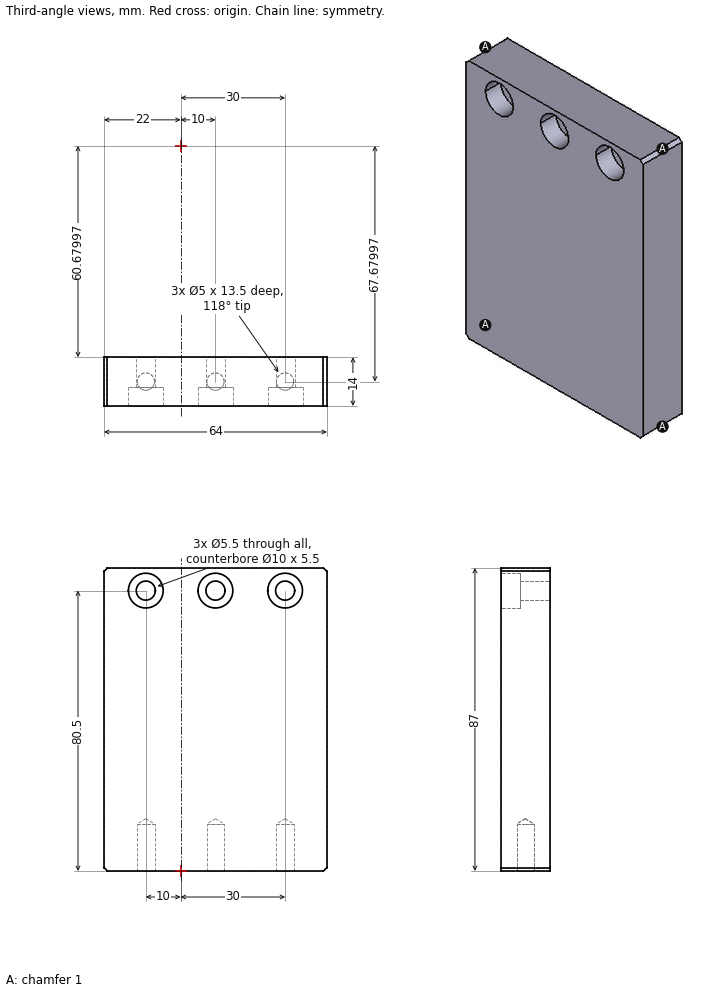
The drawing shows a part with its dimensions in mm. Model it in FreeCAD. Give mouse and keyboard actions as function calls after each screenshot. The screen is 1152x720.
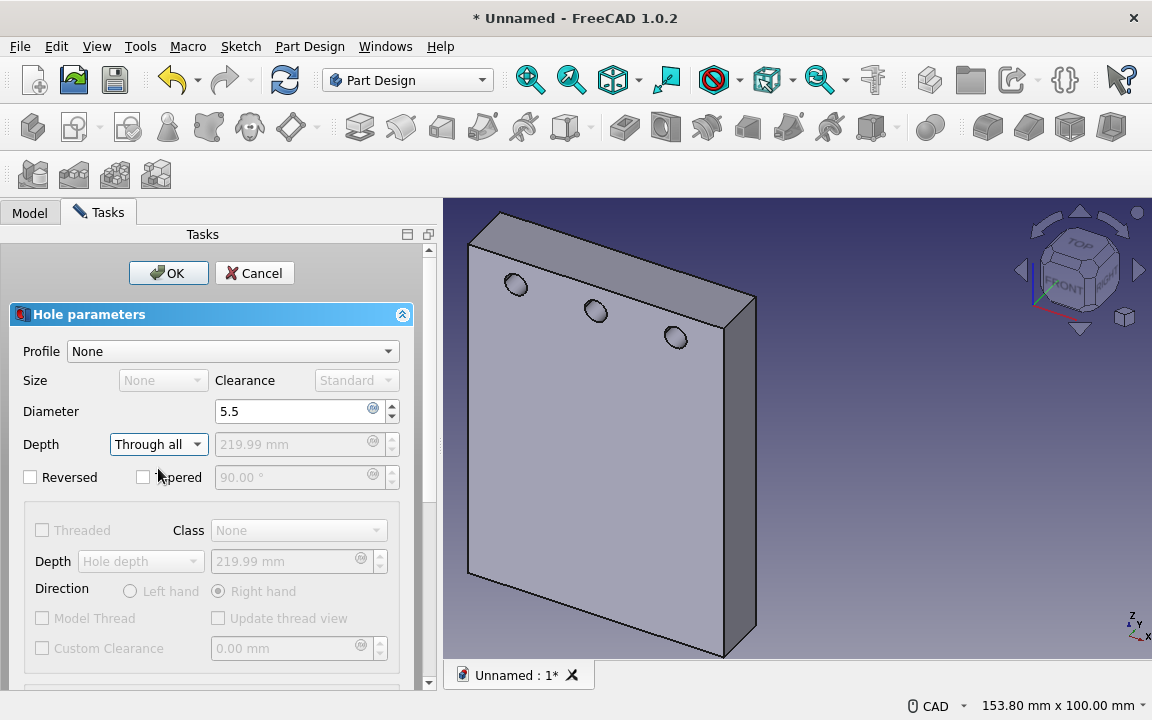
scroll(429, 467, down, 2)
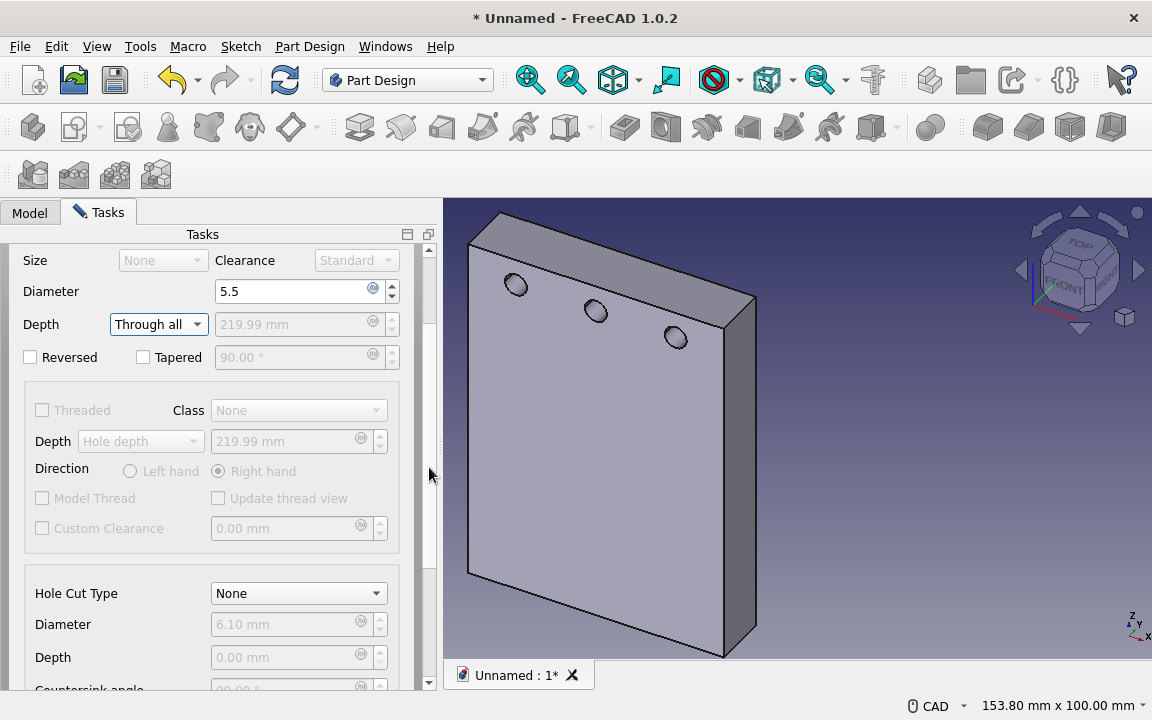
click(300, 594)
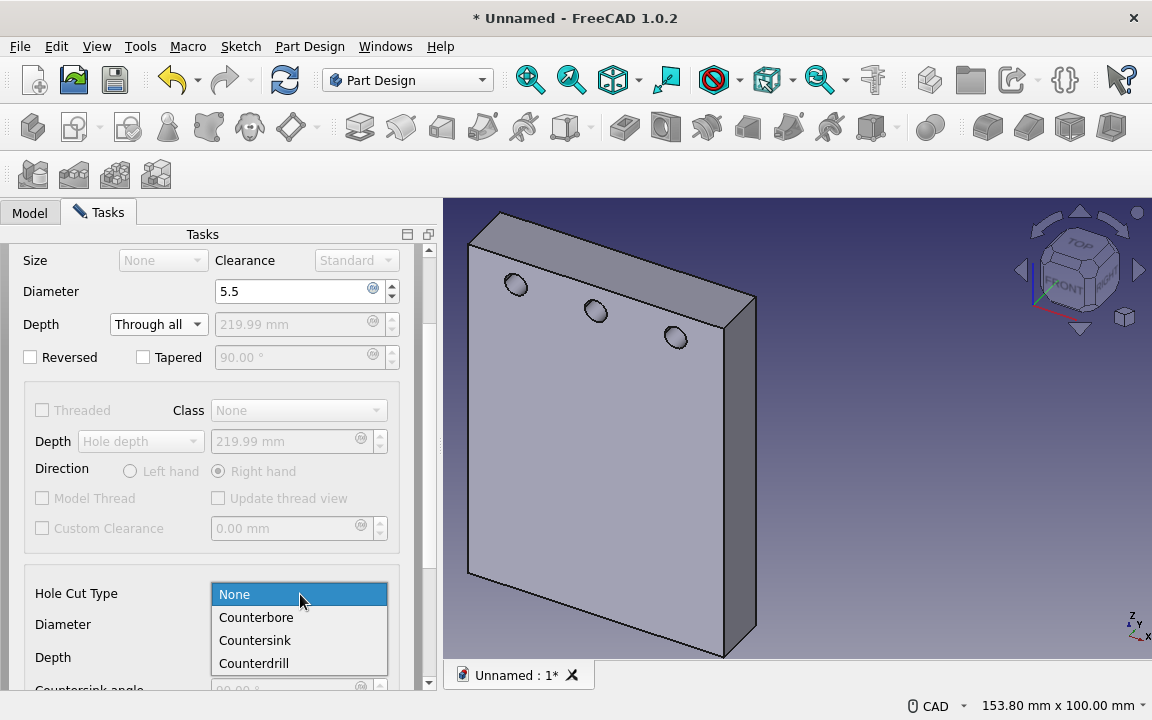
click(298, 618)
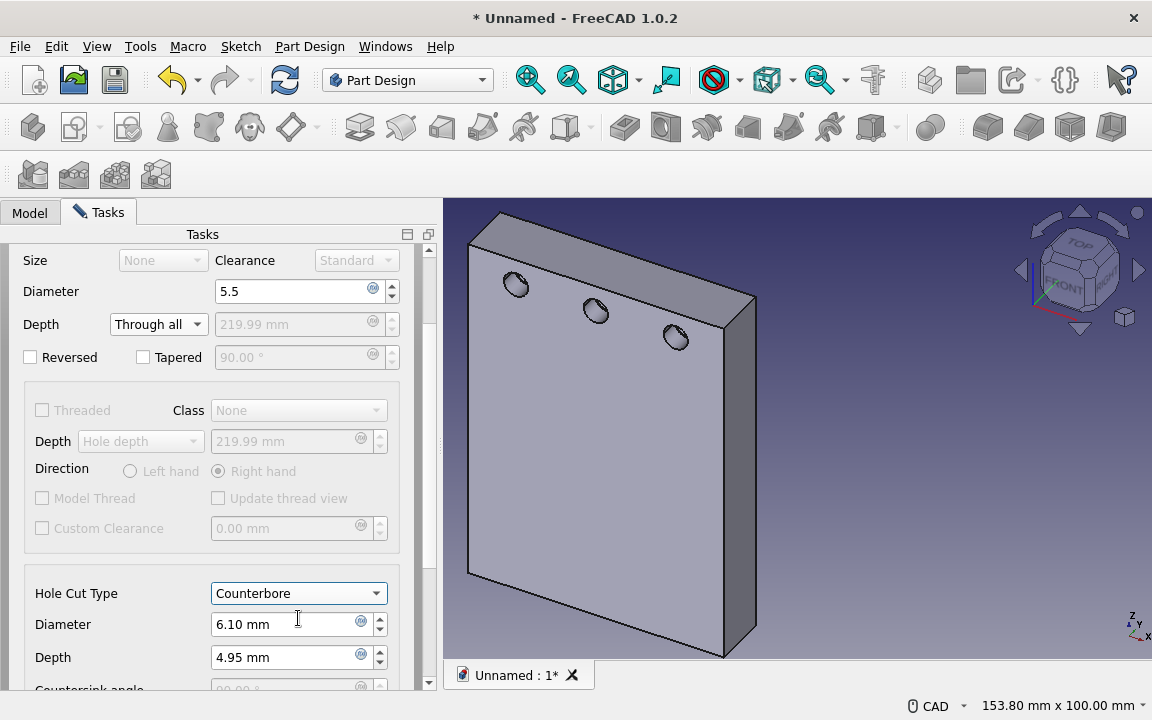
triple_click(292, 624)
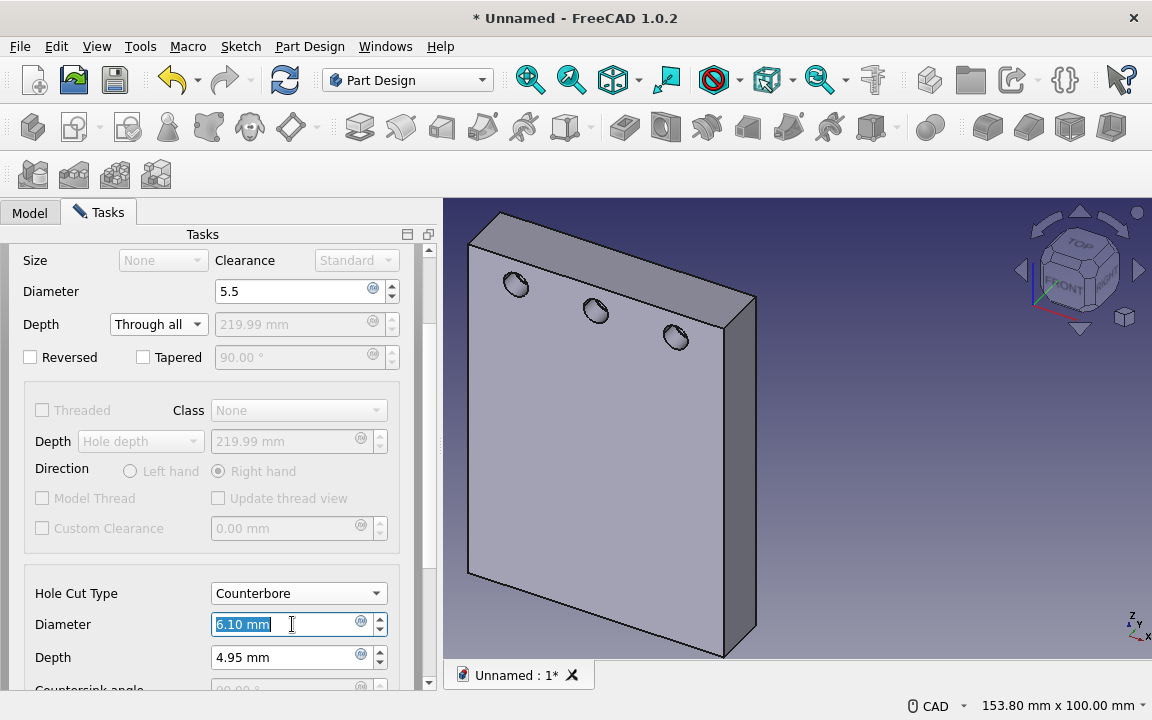
text(10)
key(Tab)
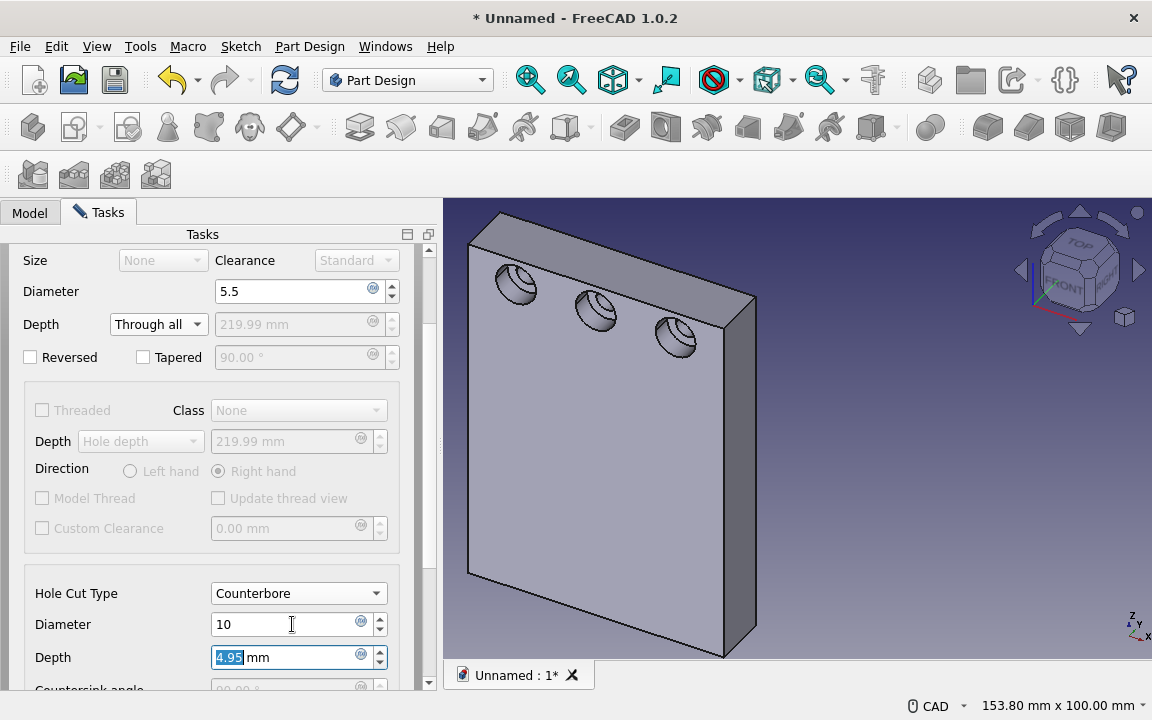
text(5.5)
key(Tab)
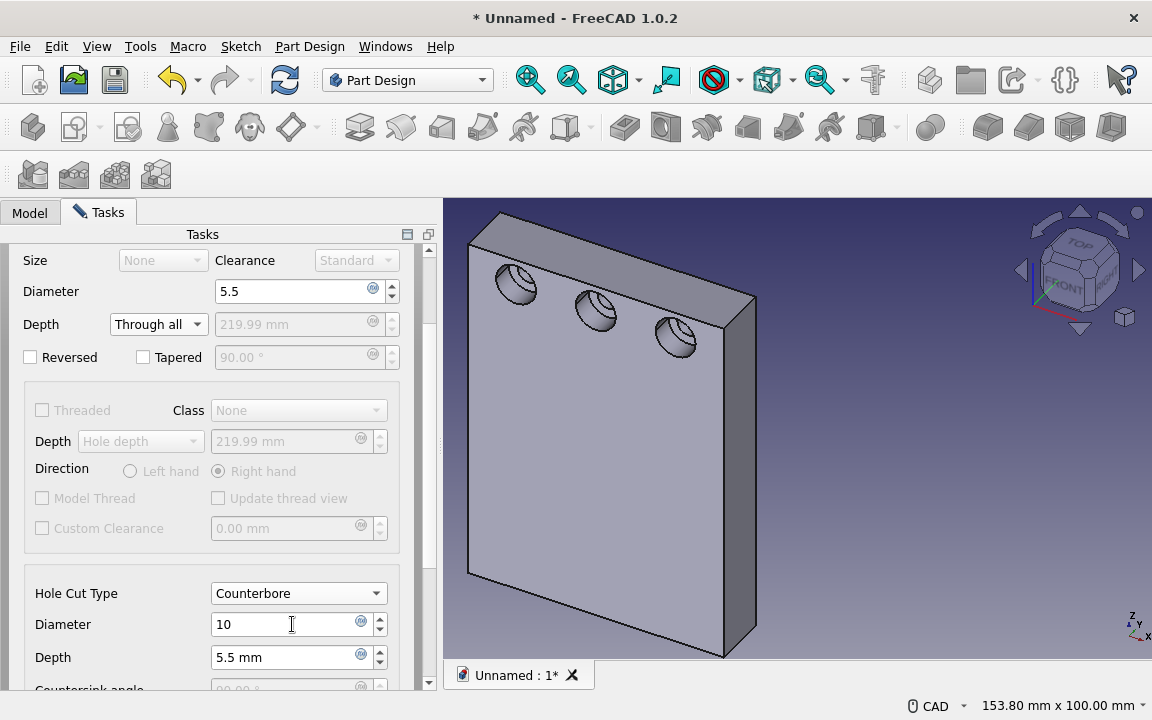
scroll(429, 467, up, 3)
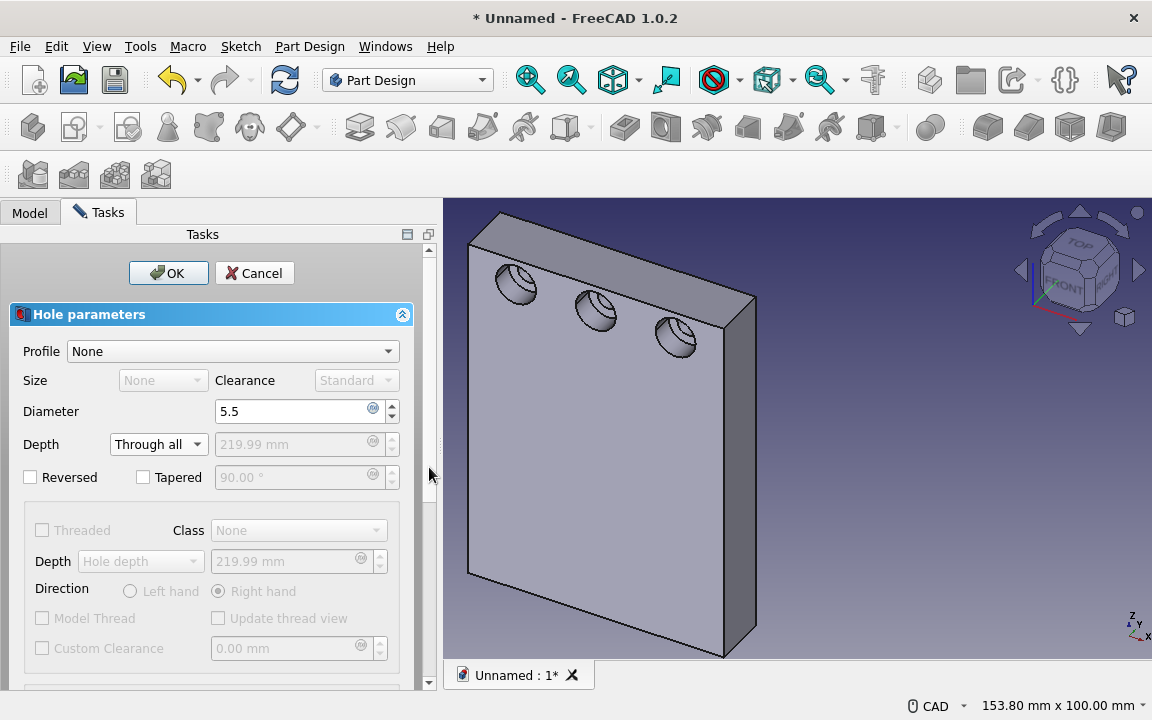
click(169, 273)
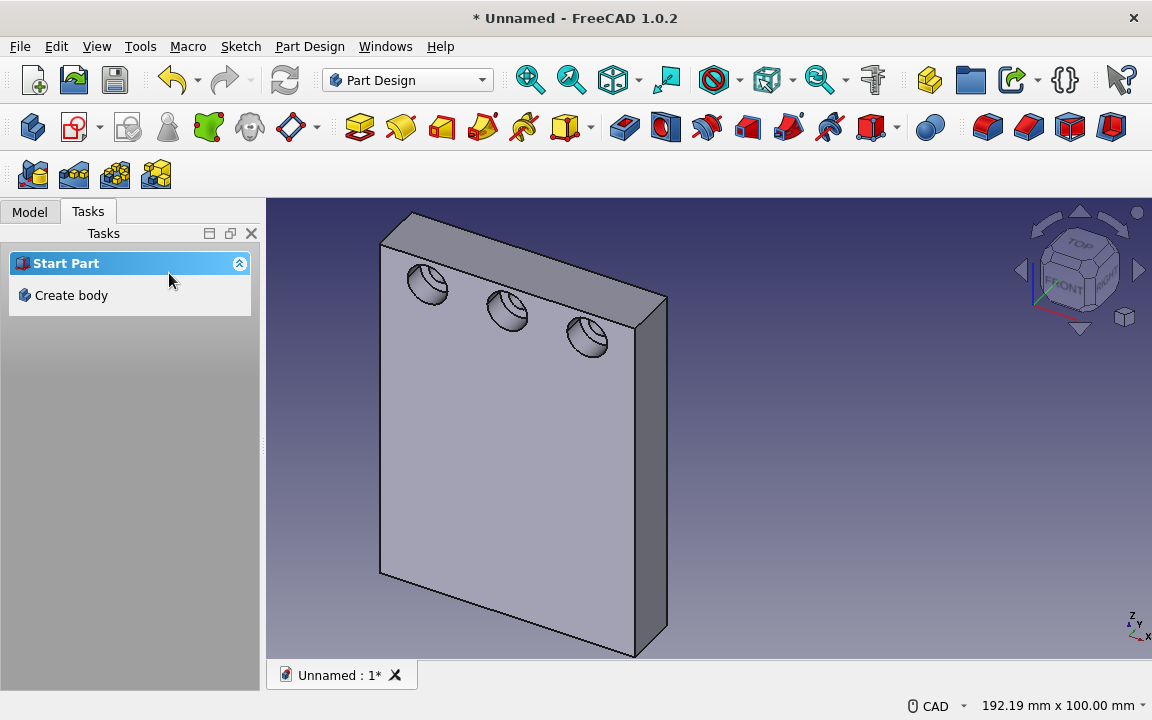
key(5)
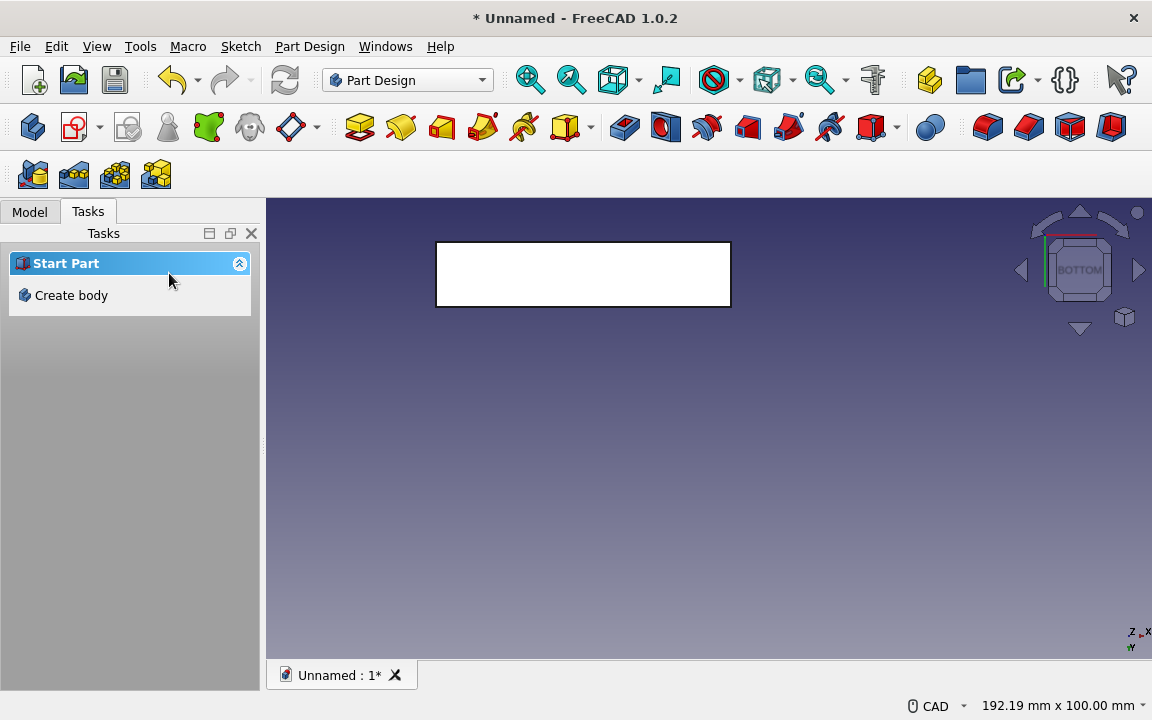
key(v)
key(f)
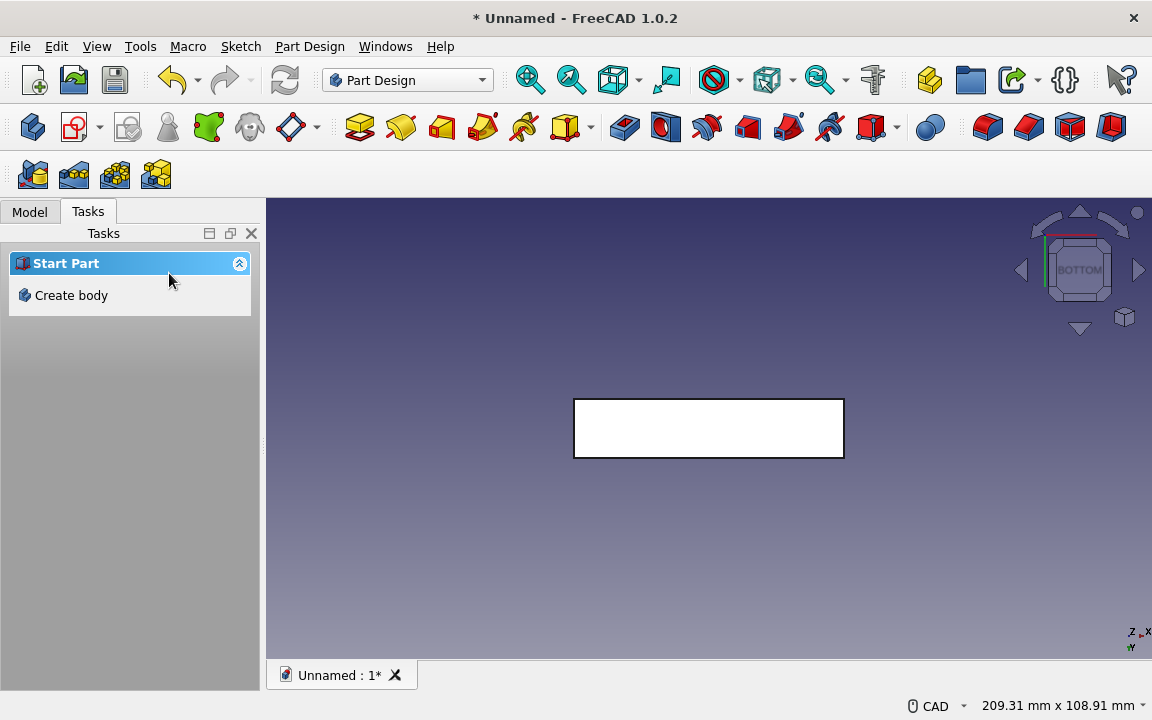
click(786, 427)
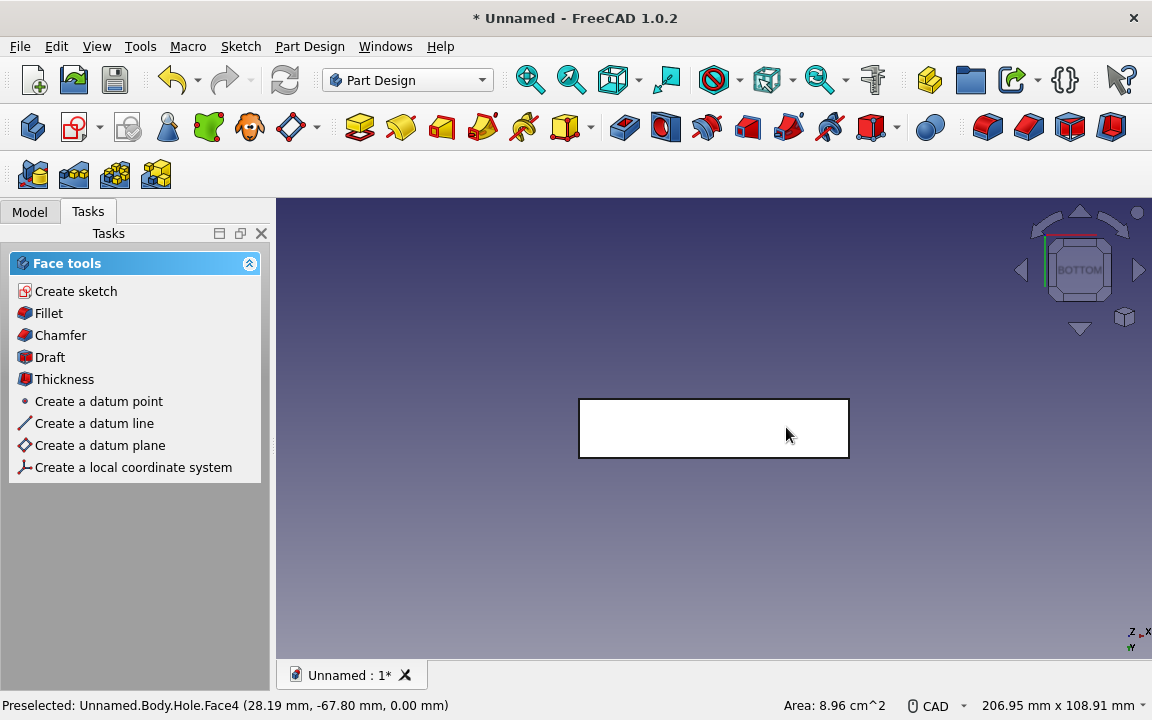
click(74, 128)